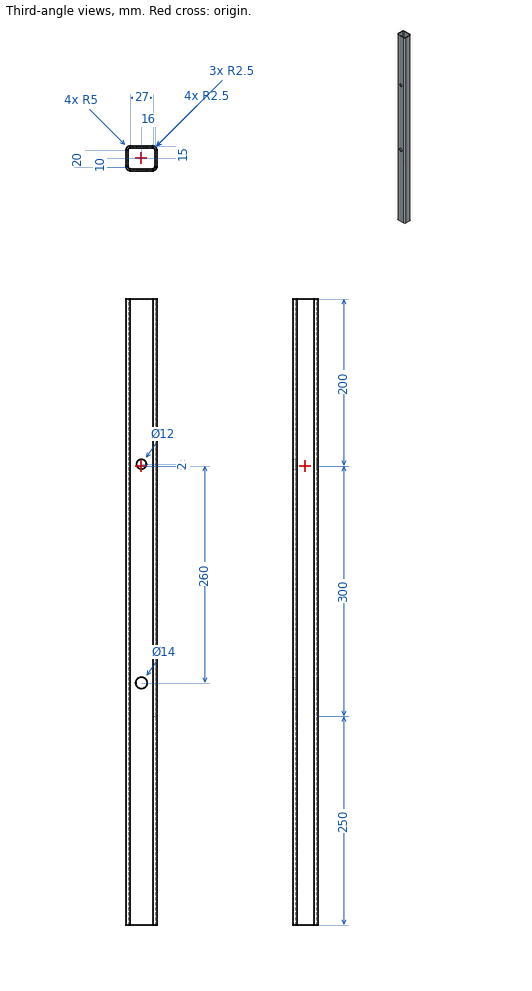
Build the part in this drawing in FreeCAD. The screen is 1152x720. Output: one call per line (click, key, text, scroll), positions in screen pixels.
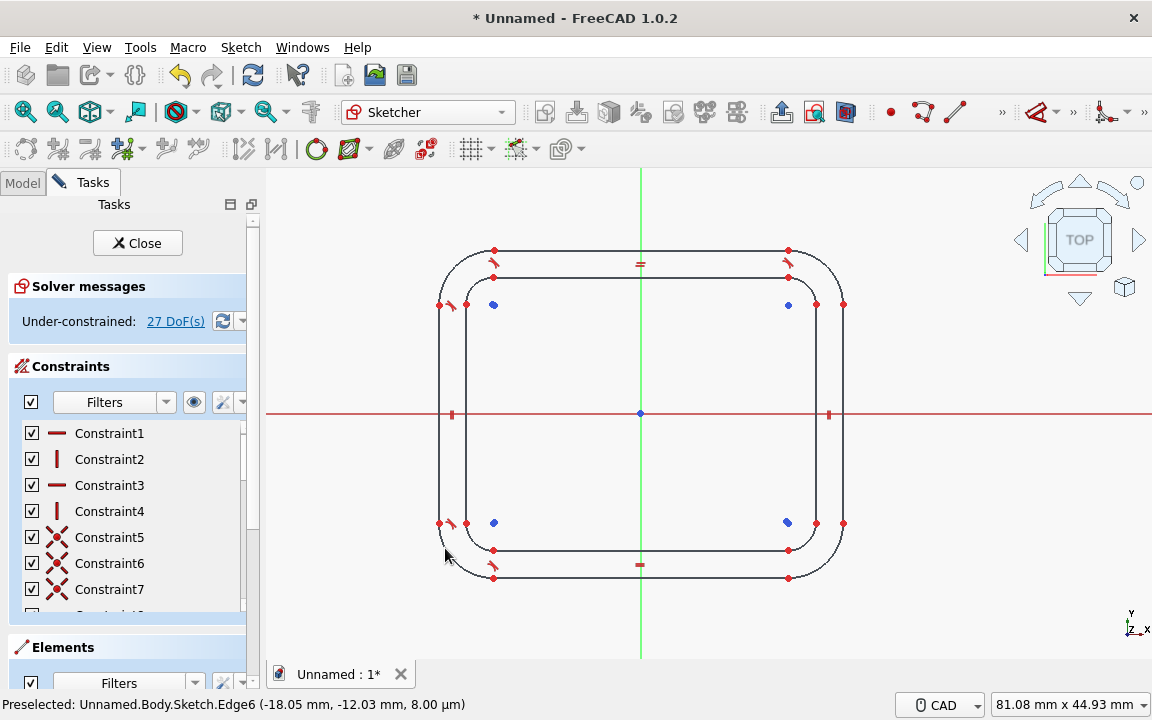
click(582, 578)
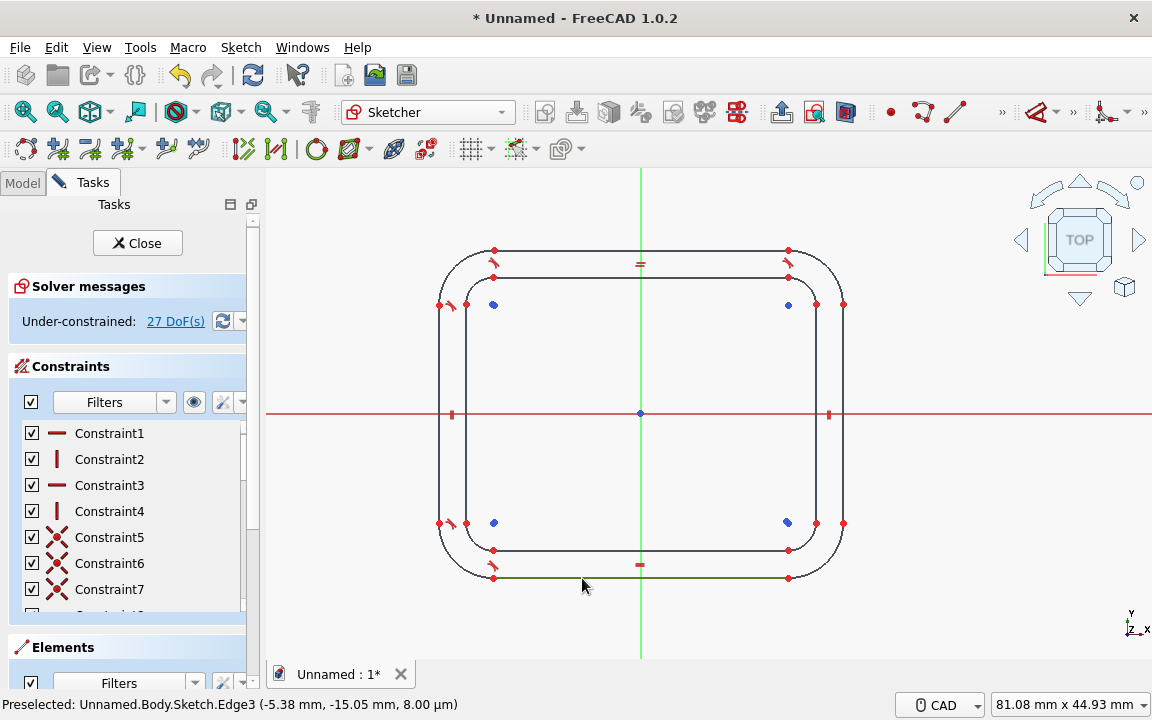
click(813, 572)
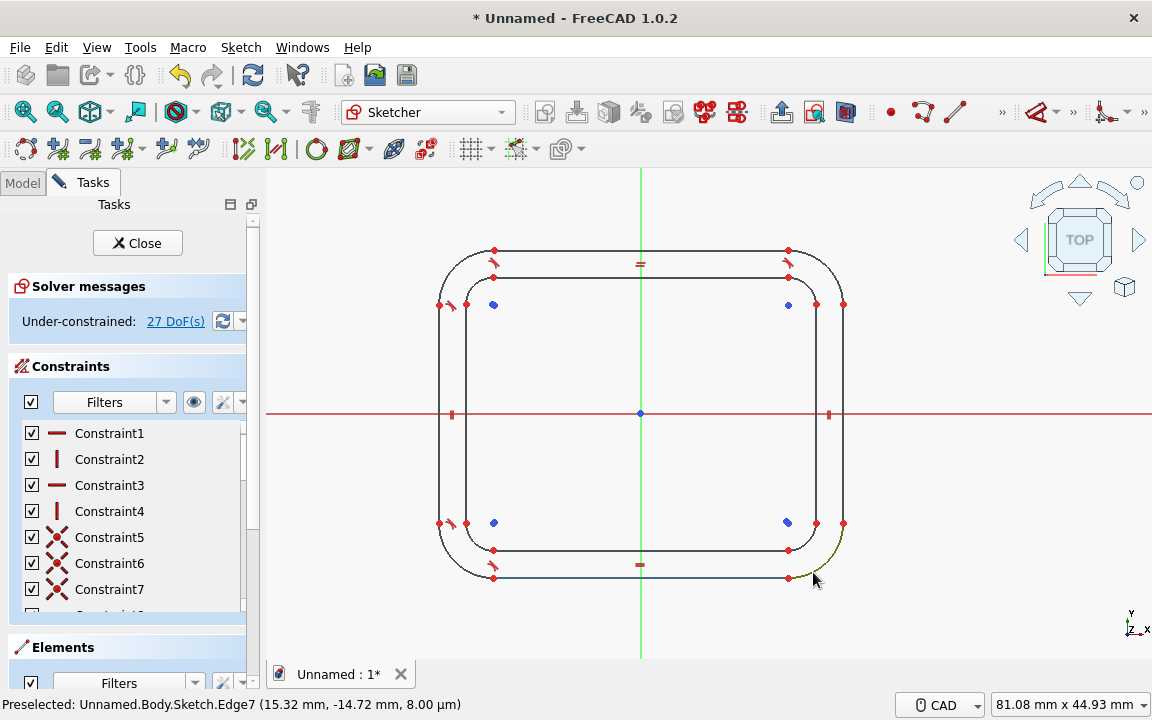
key(t)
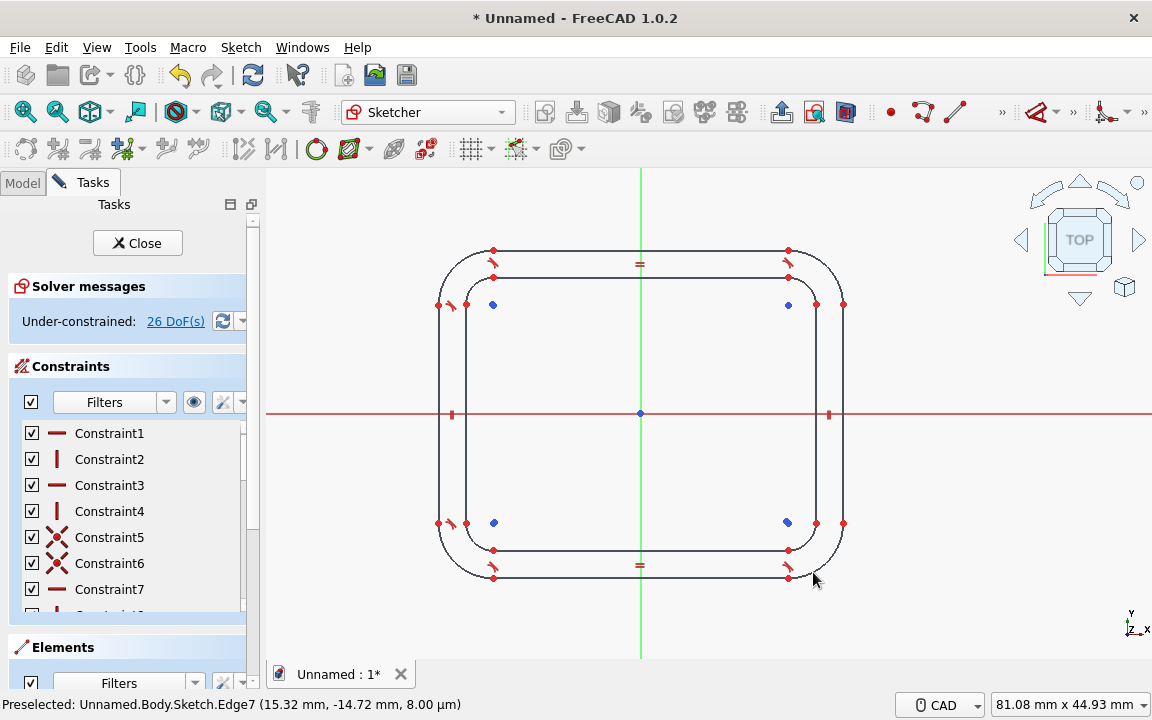
click(843, 458)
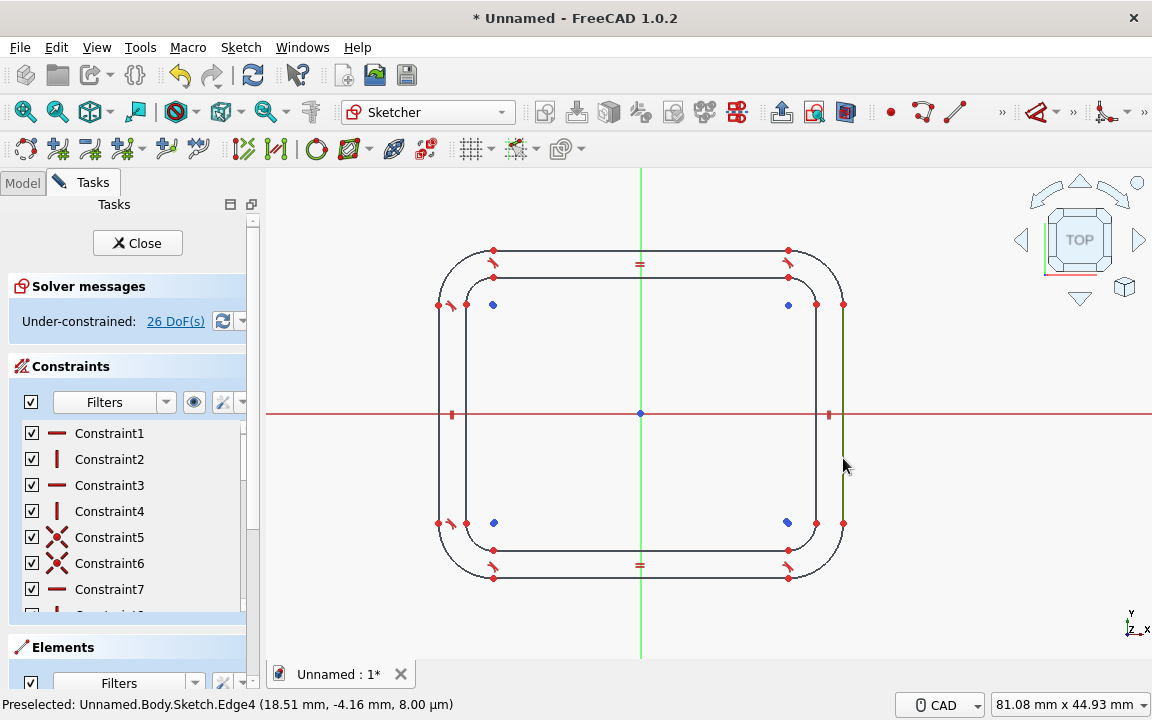
click(813, 572)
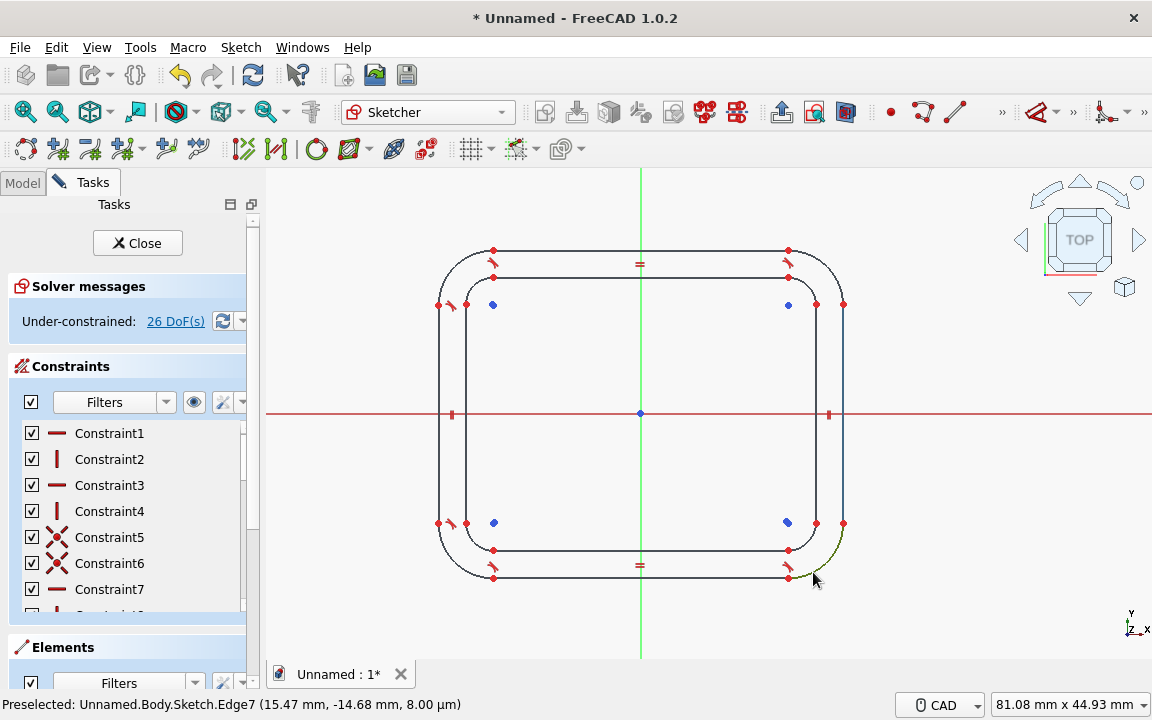
key(t)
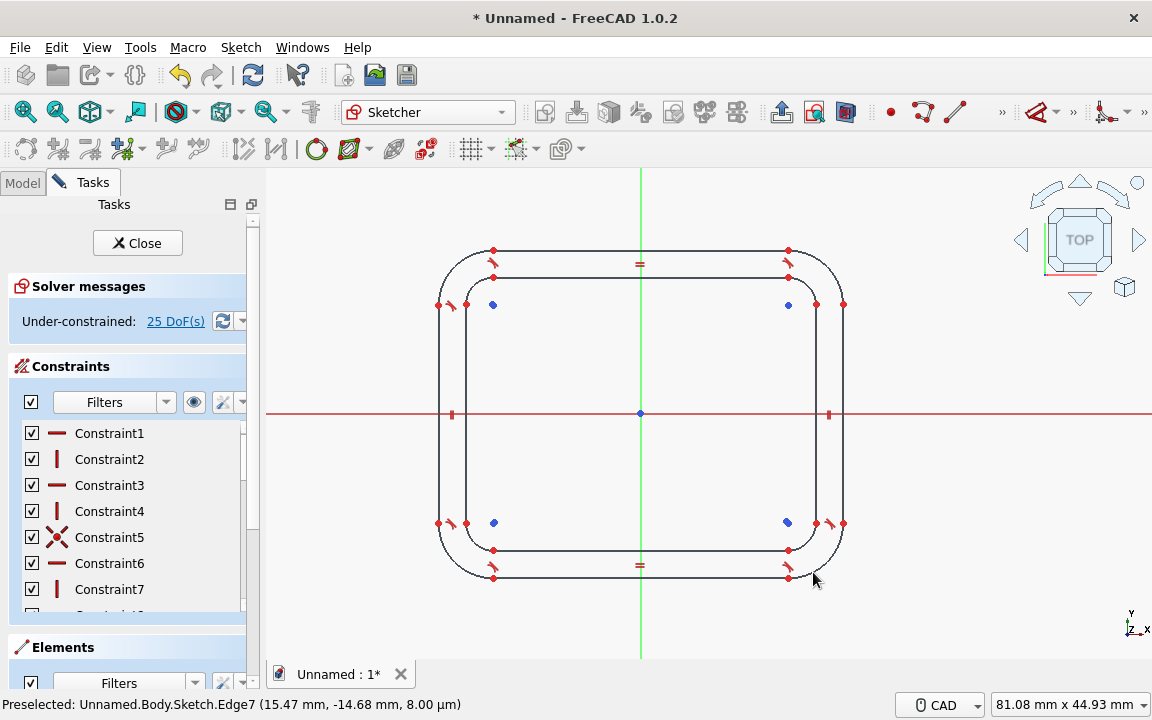
click(843, 458)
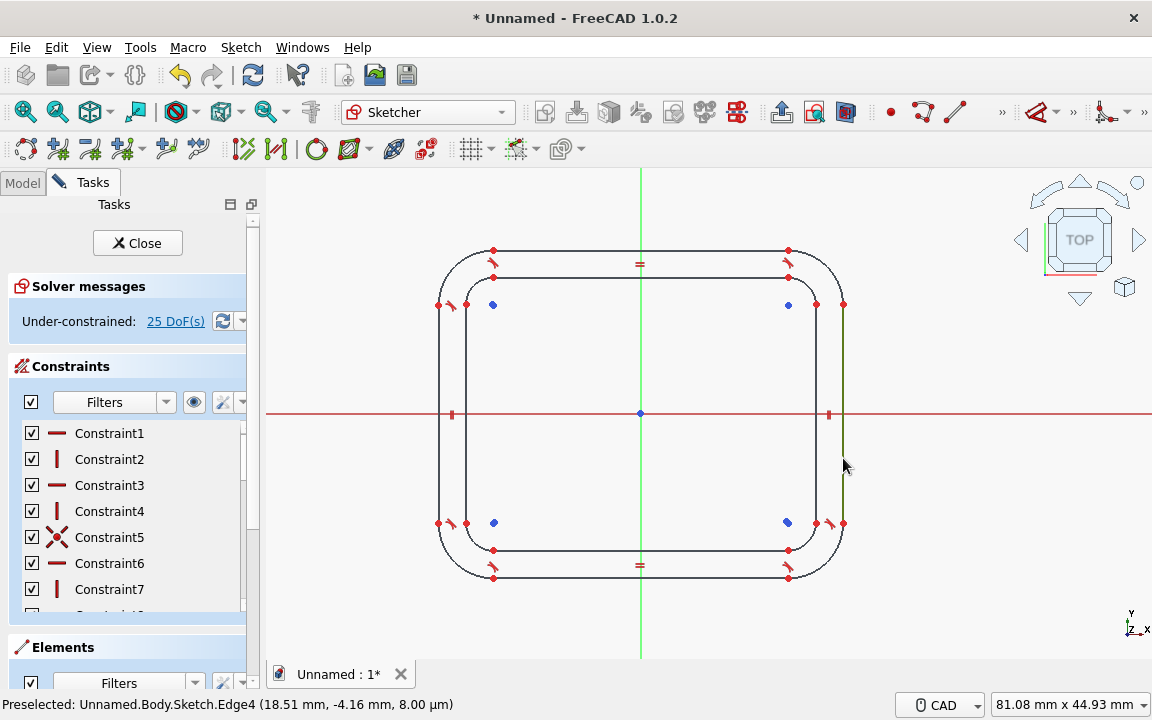
click(837, 280)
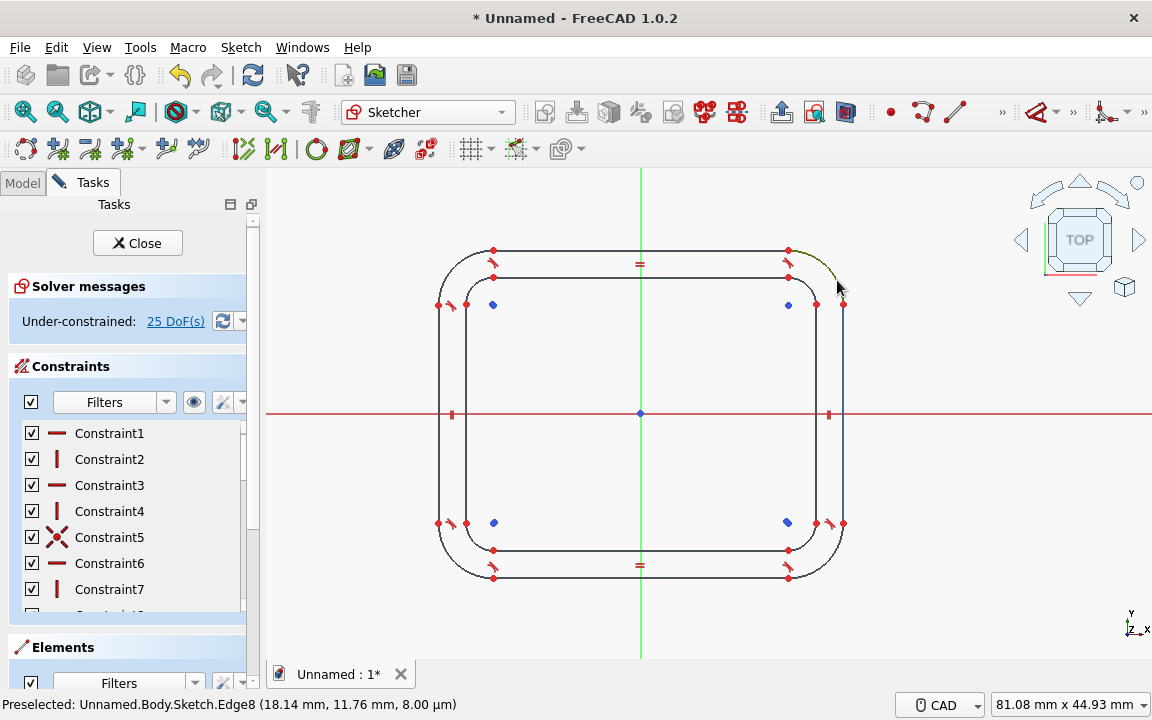
key(t)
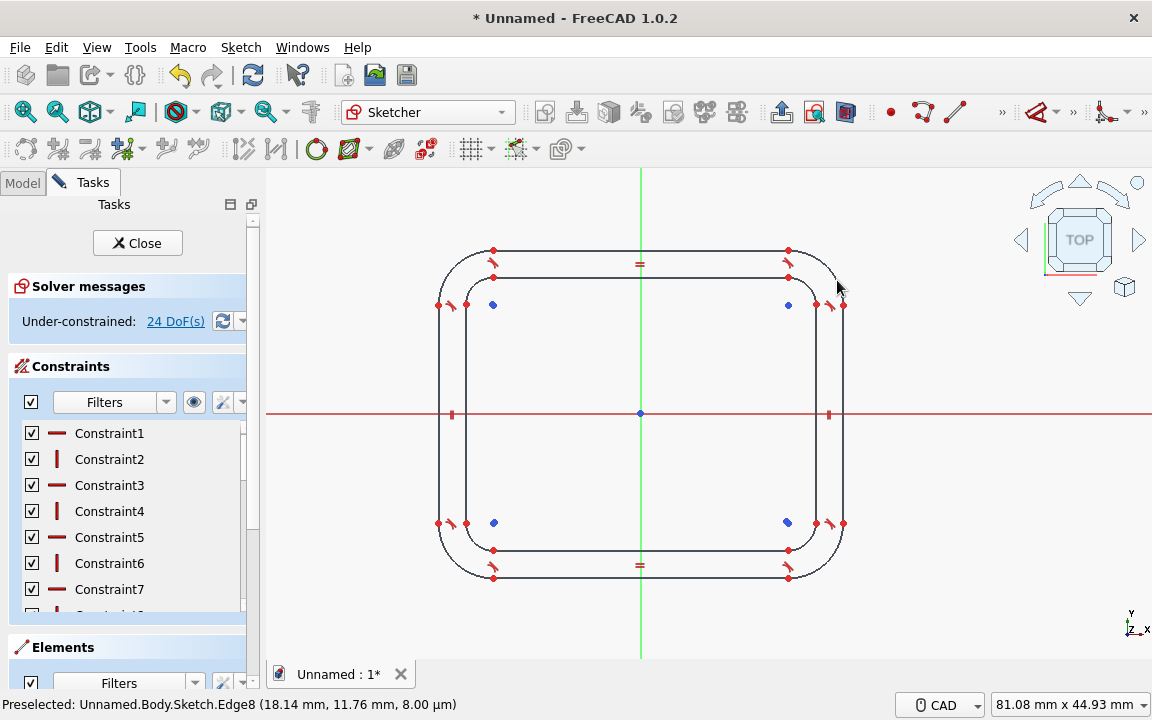
click(582, 278)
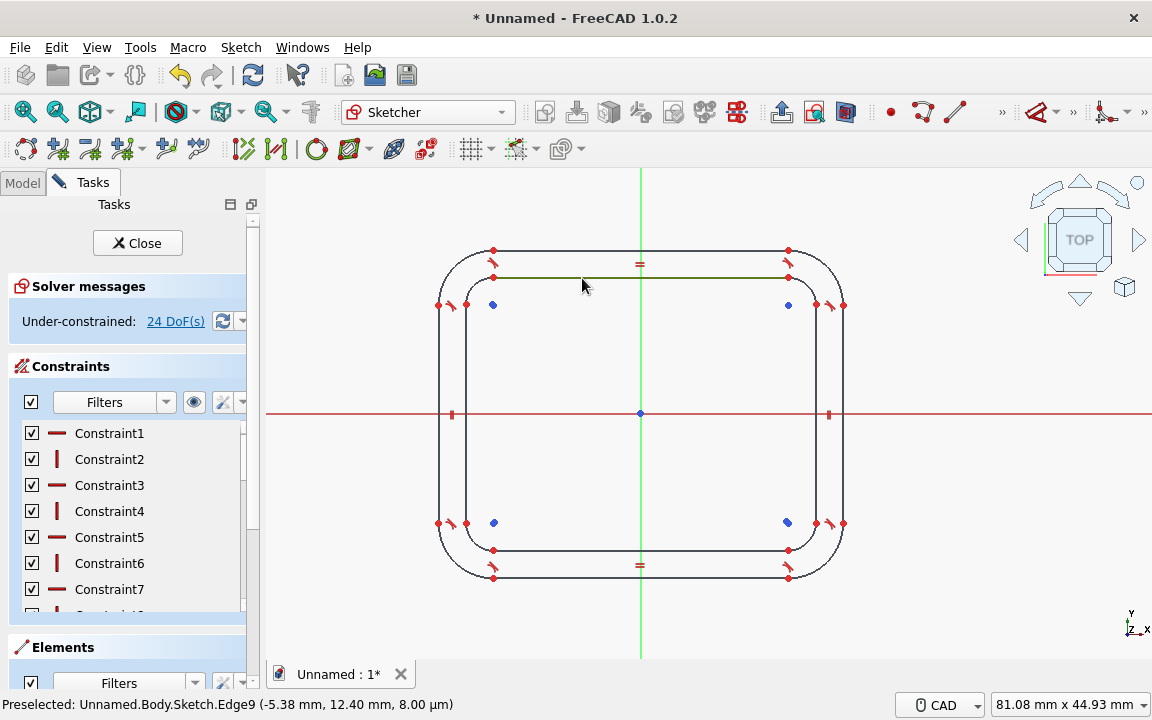
click(813, 293)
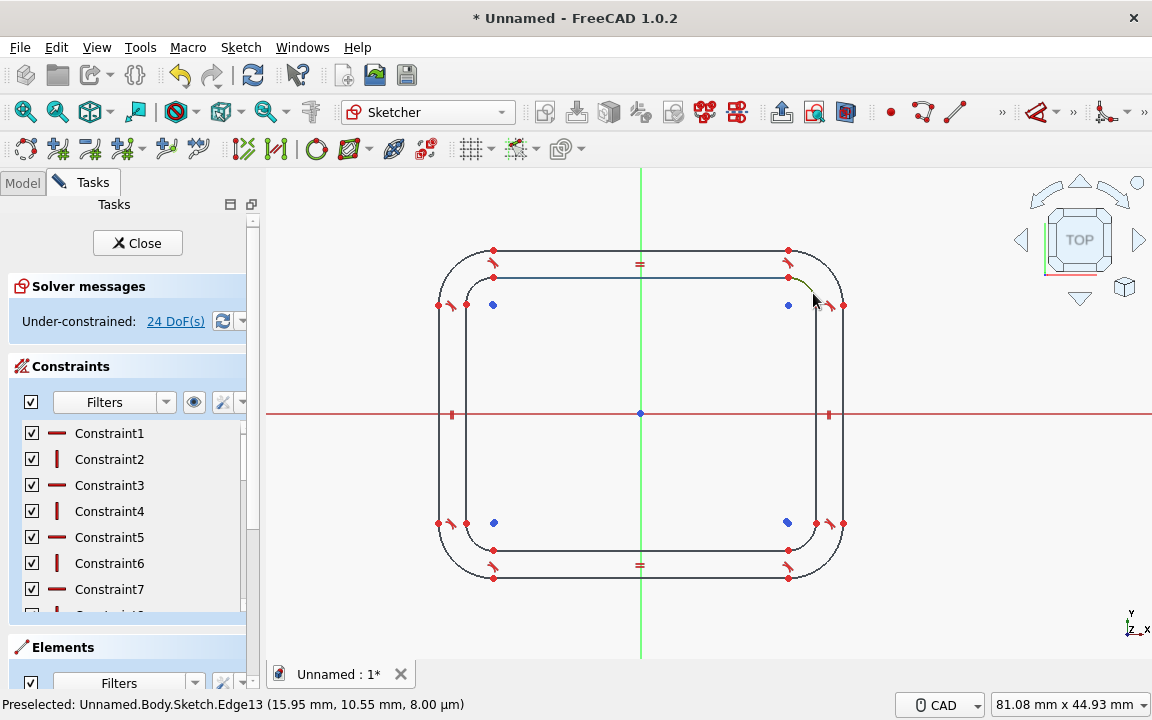
key(t)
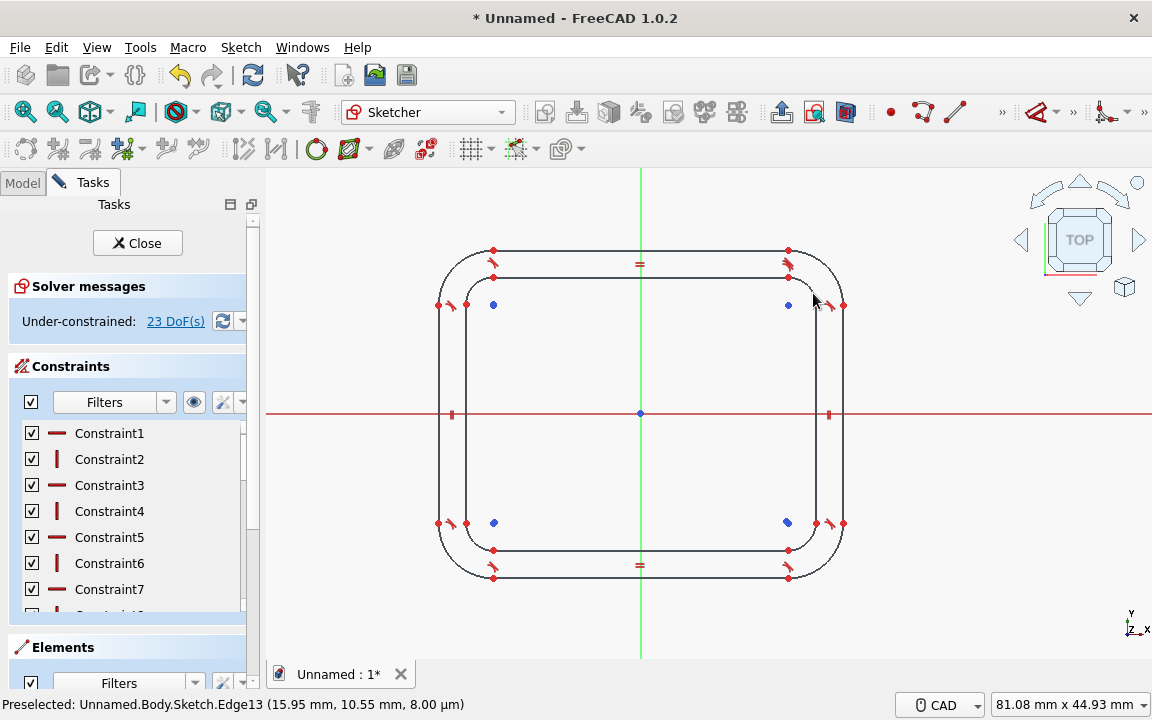
click(582, 278)